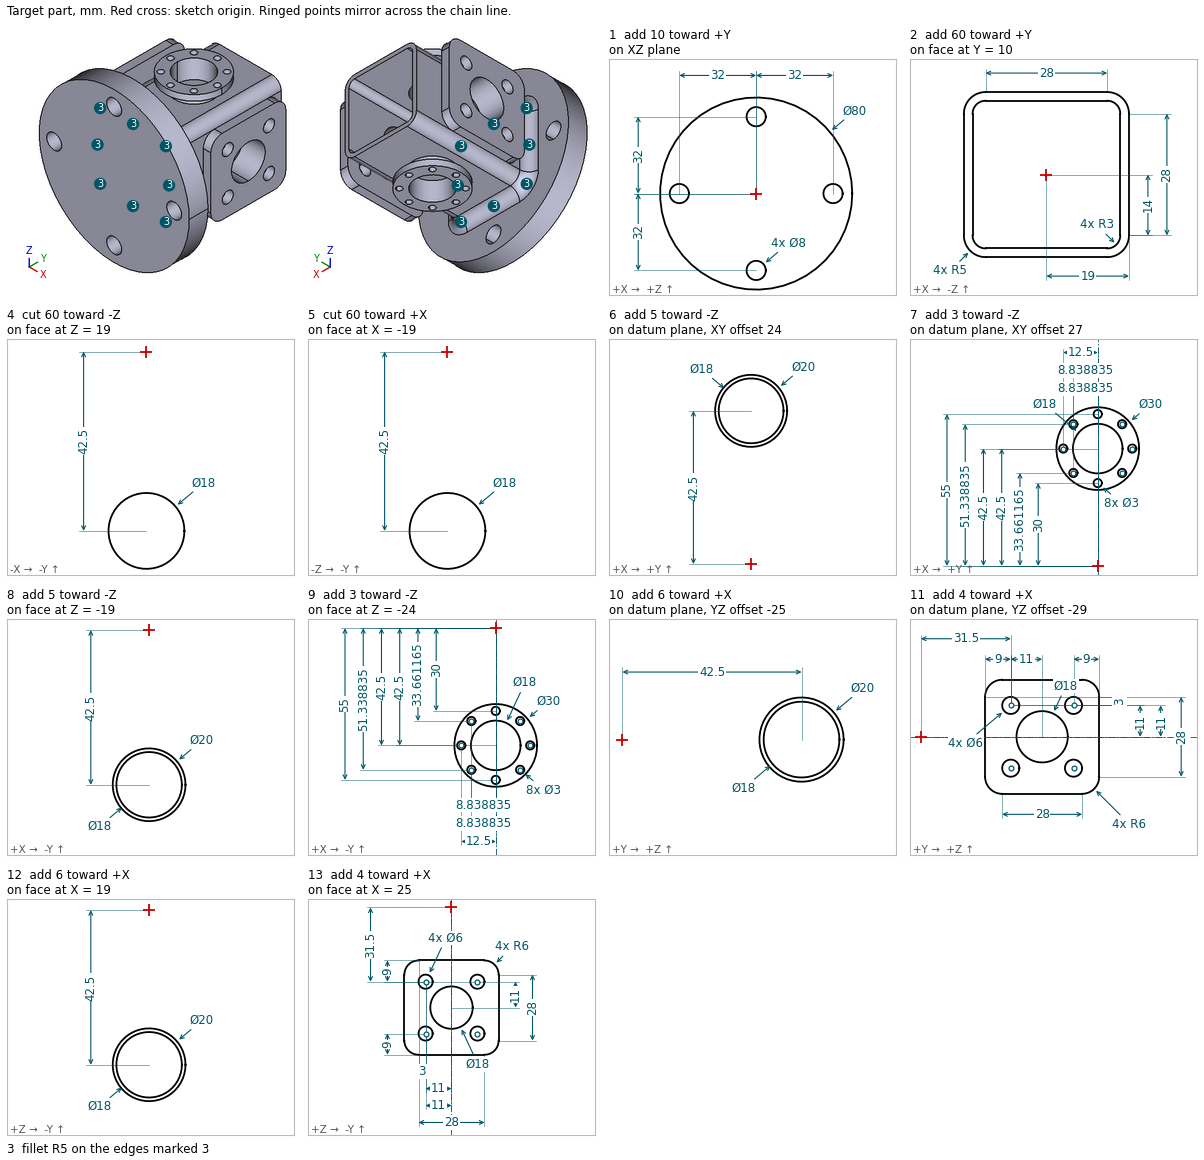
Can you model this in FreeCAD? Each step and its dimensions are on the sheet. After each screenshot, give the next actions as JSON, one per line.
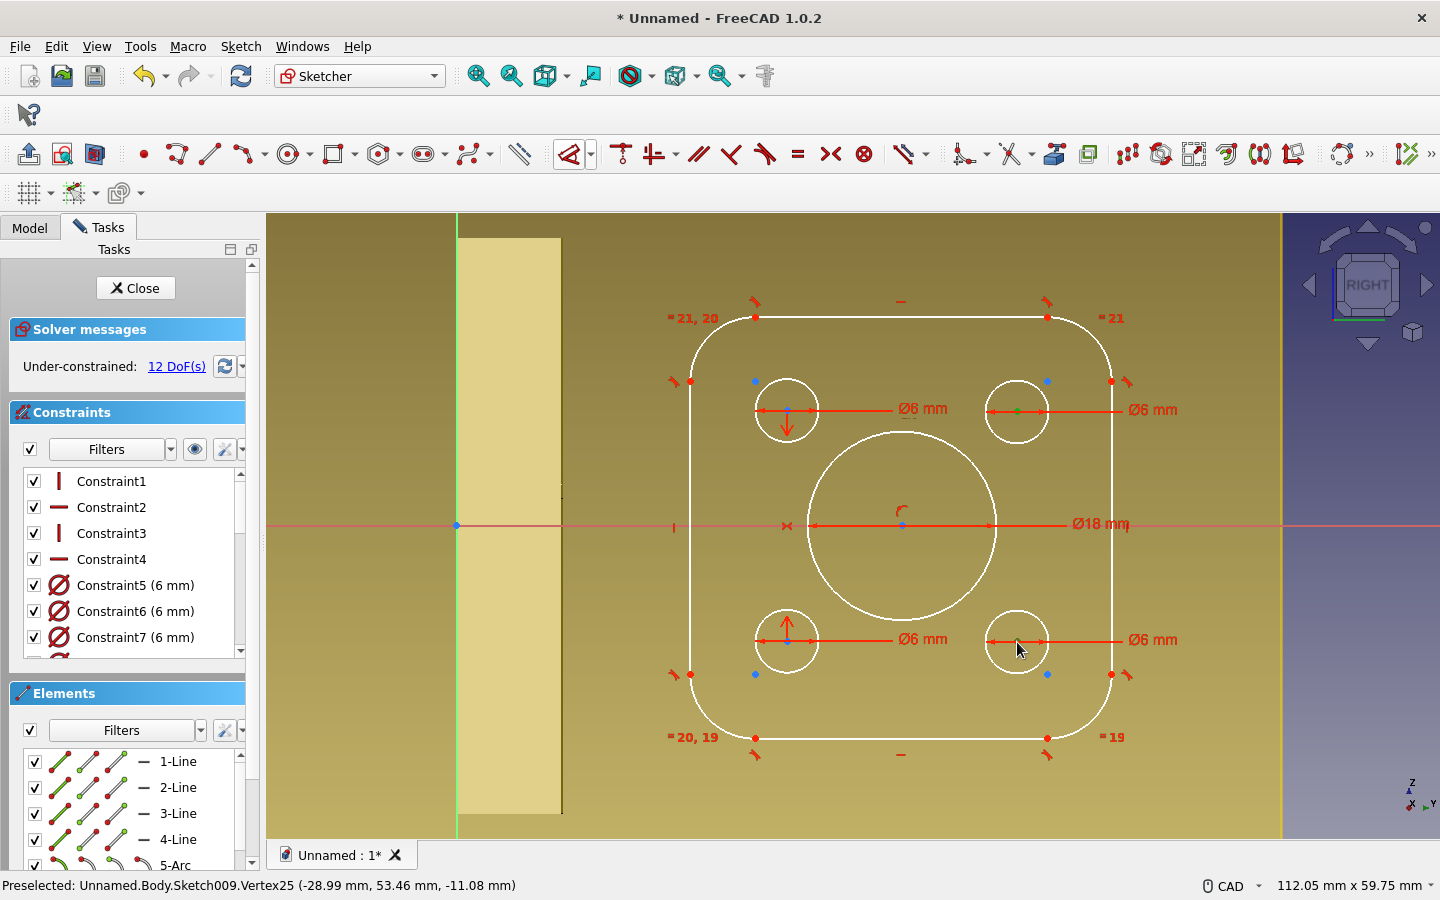
{"action": "left_click", "coordinate": [364, 526]}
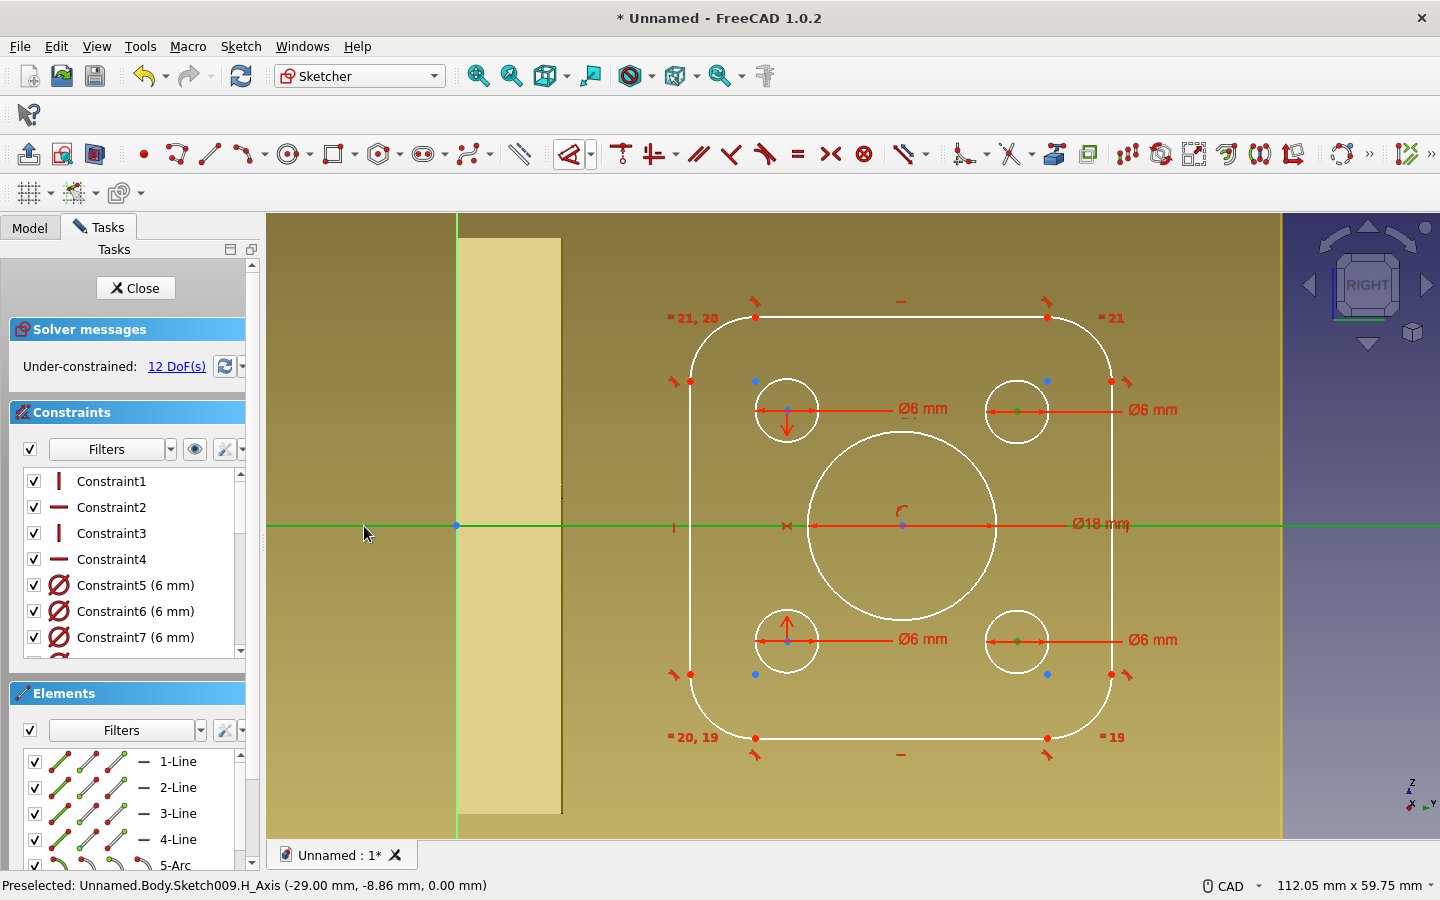
{"action": "key", "text": "s"}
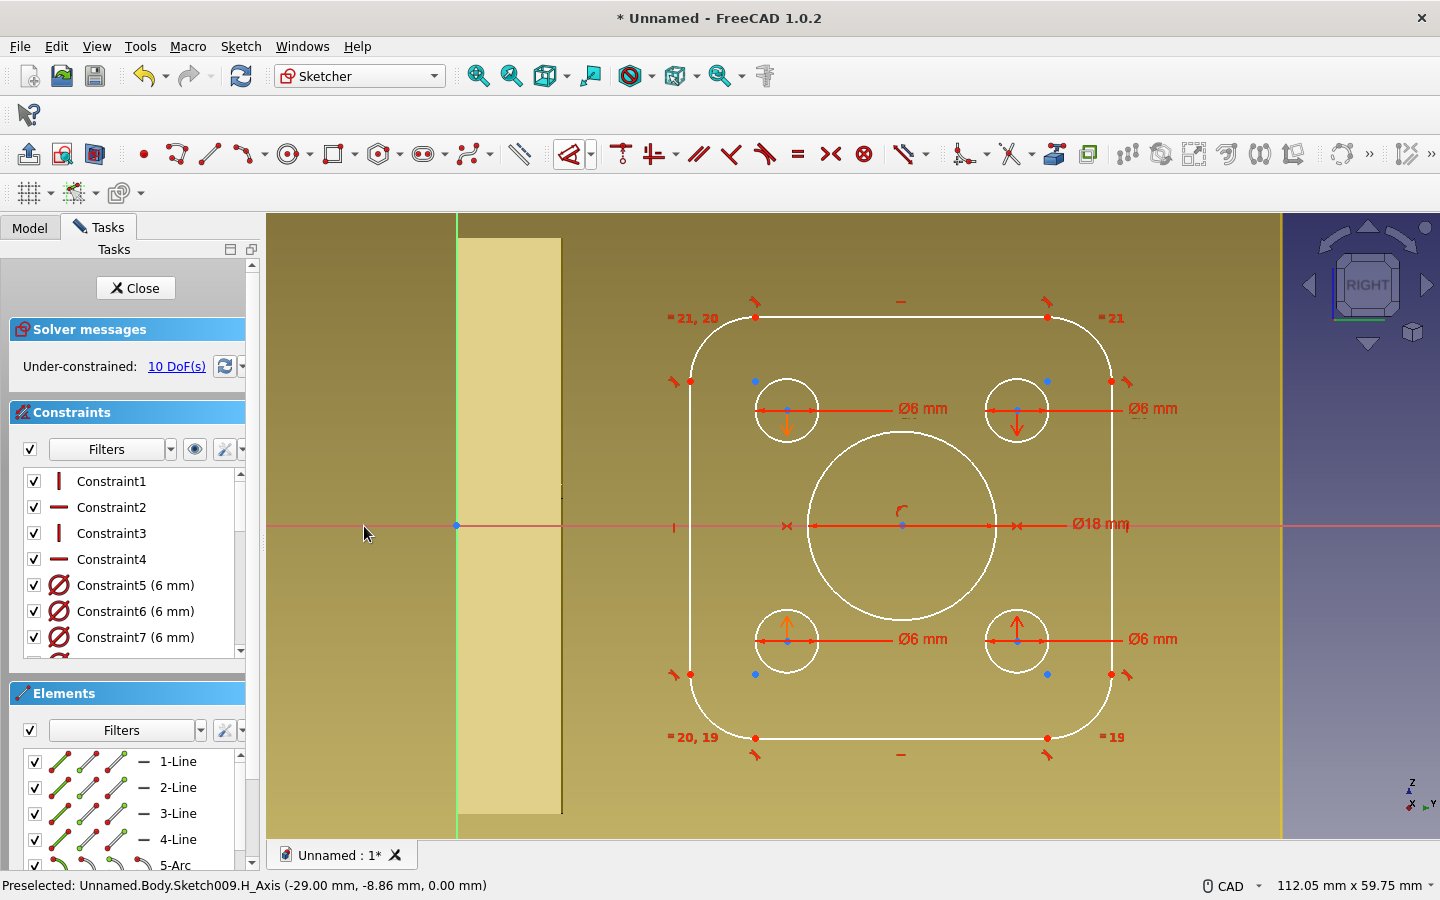
{"action": "left_click", "coordinate": [1076, 732]}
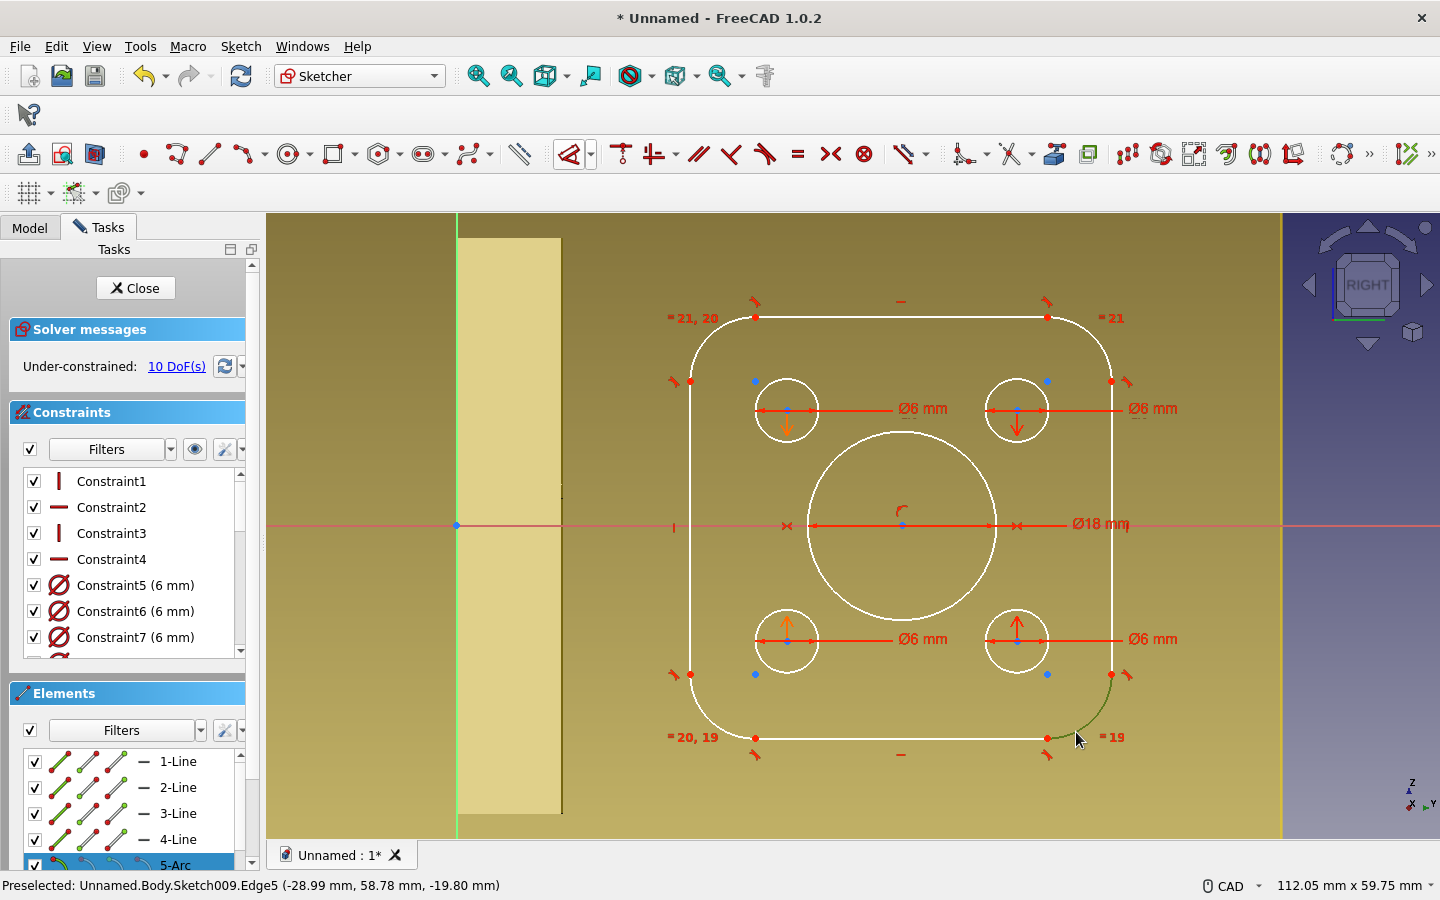
{"action": "key", "text": "k r"}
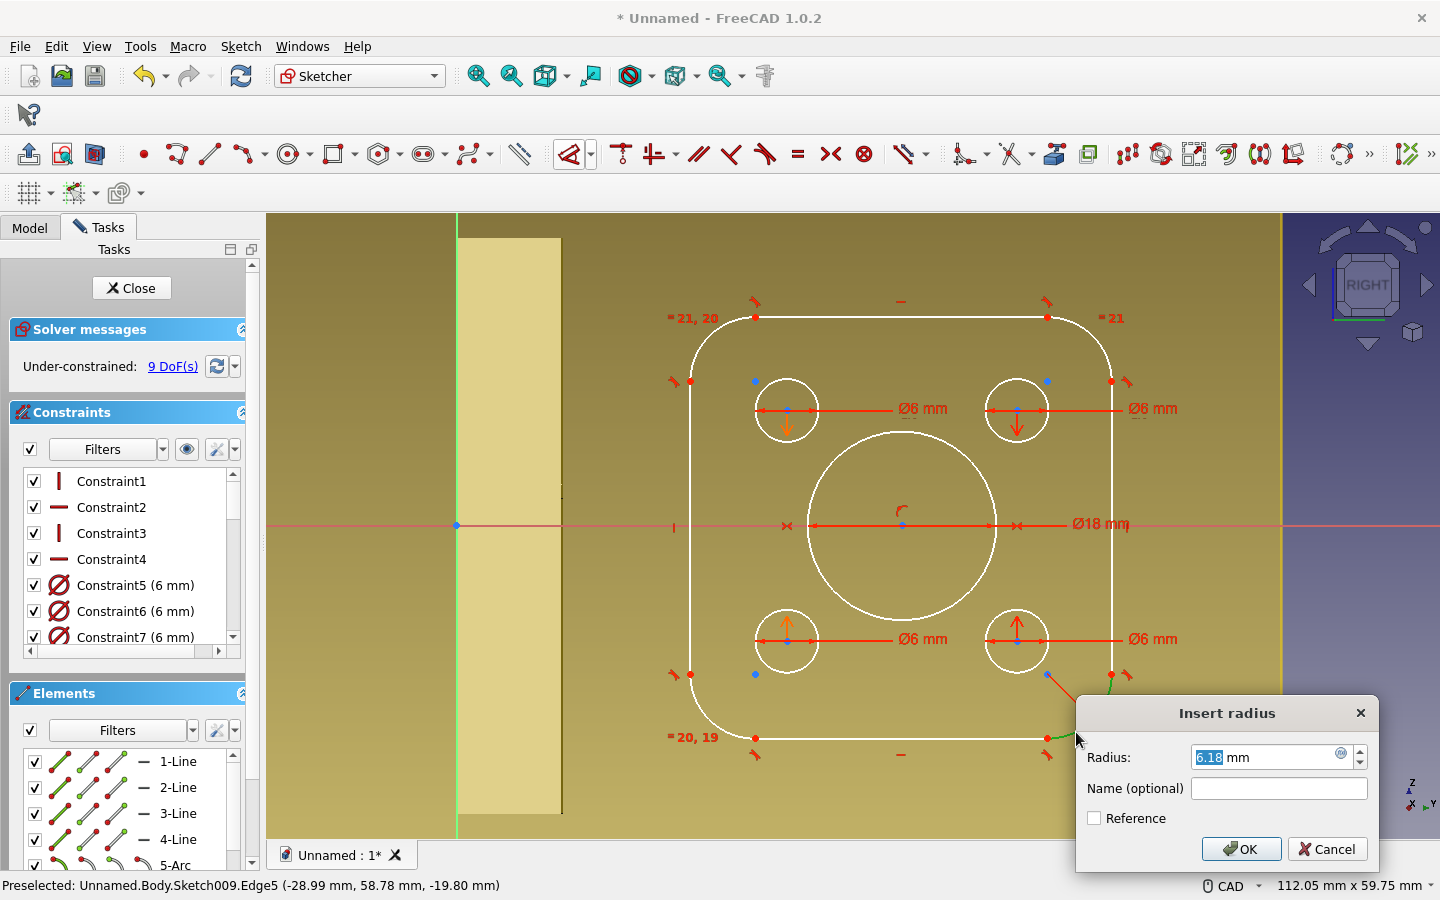
{"action": "type", "text": "6"}
{"action": "key", "text": "Return"}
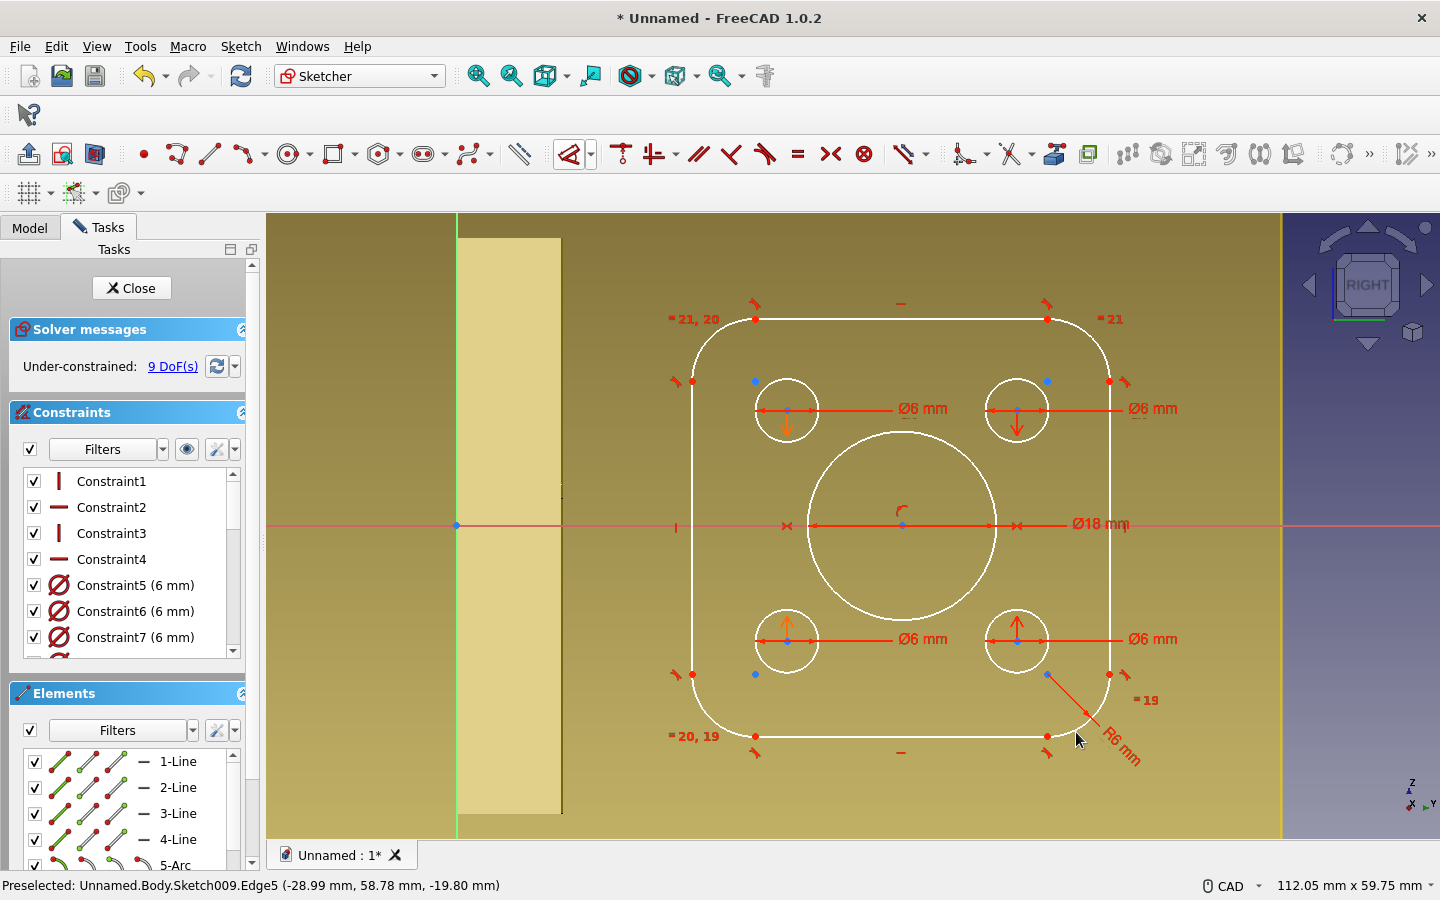
{"action": "left_click", "coordinate": [1110, 470]}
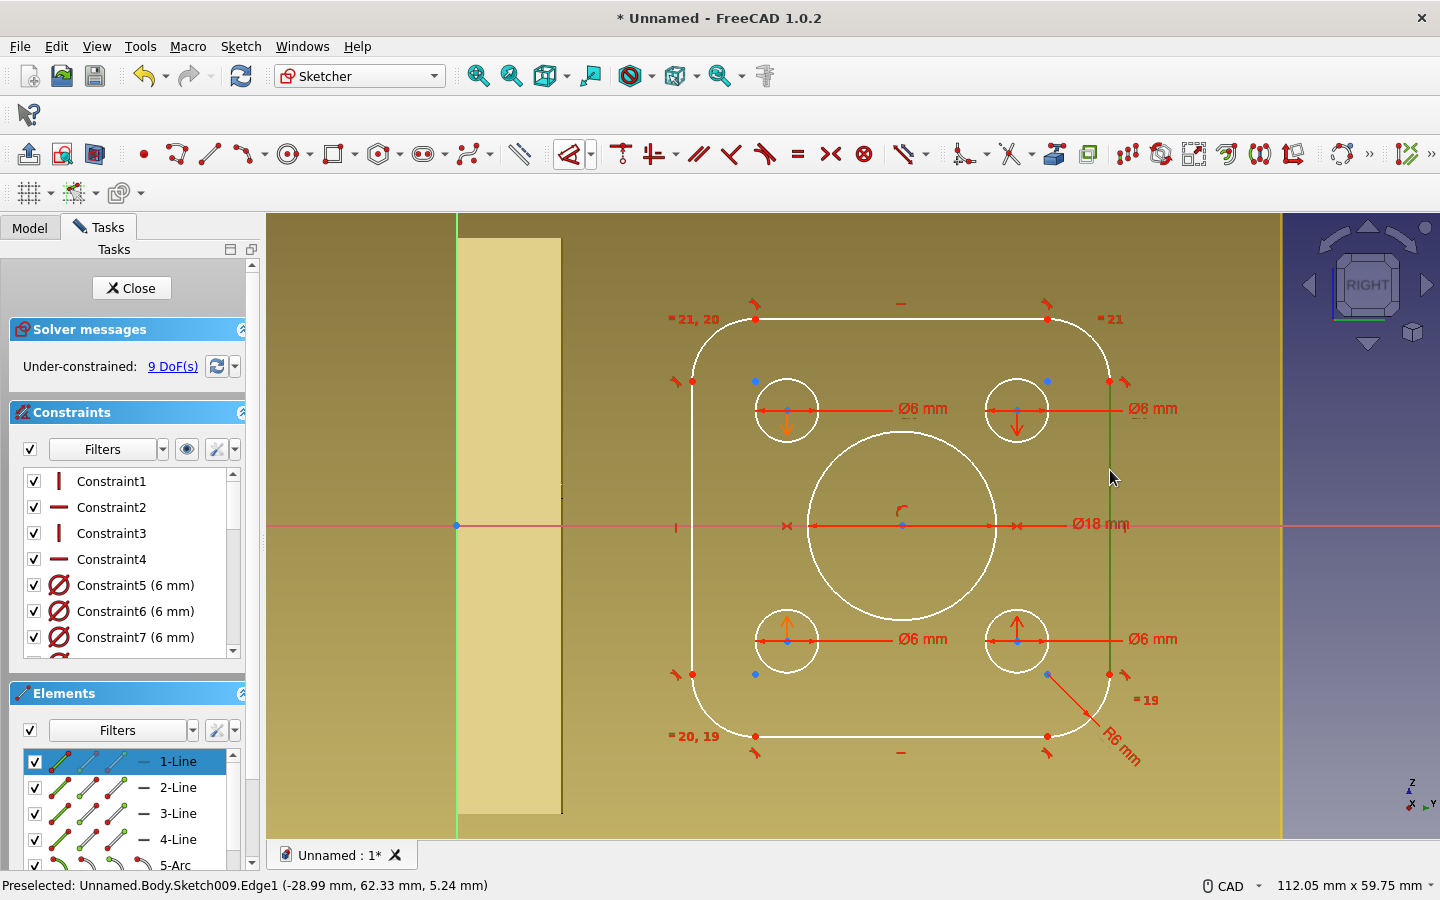
{"action": "left_click", "coordinate": [590, 154]}